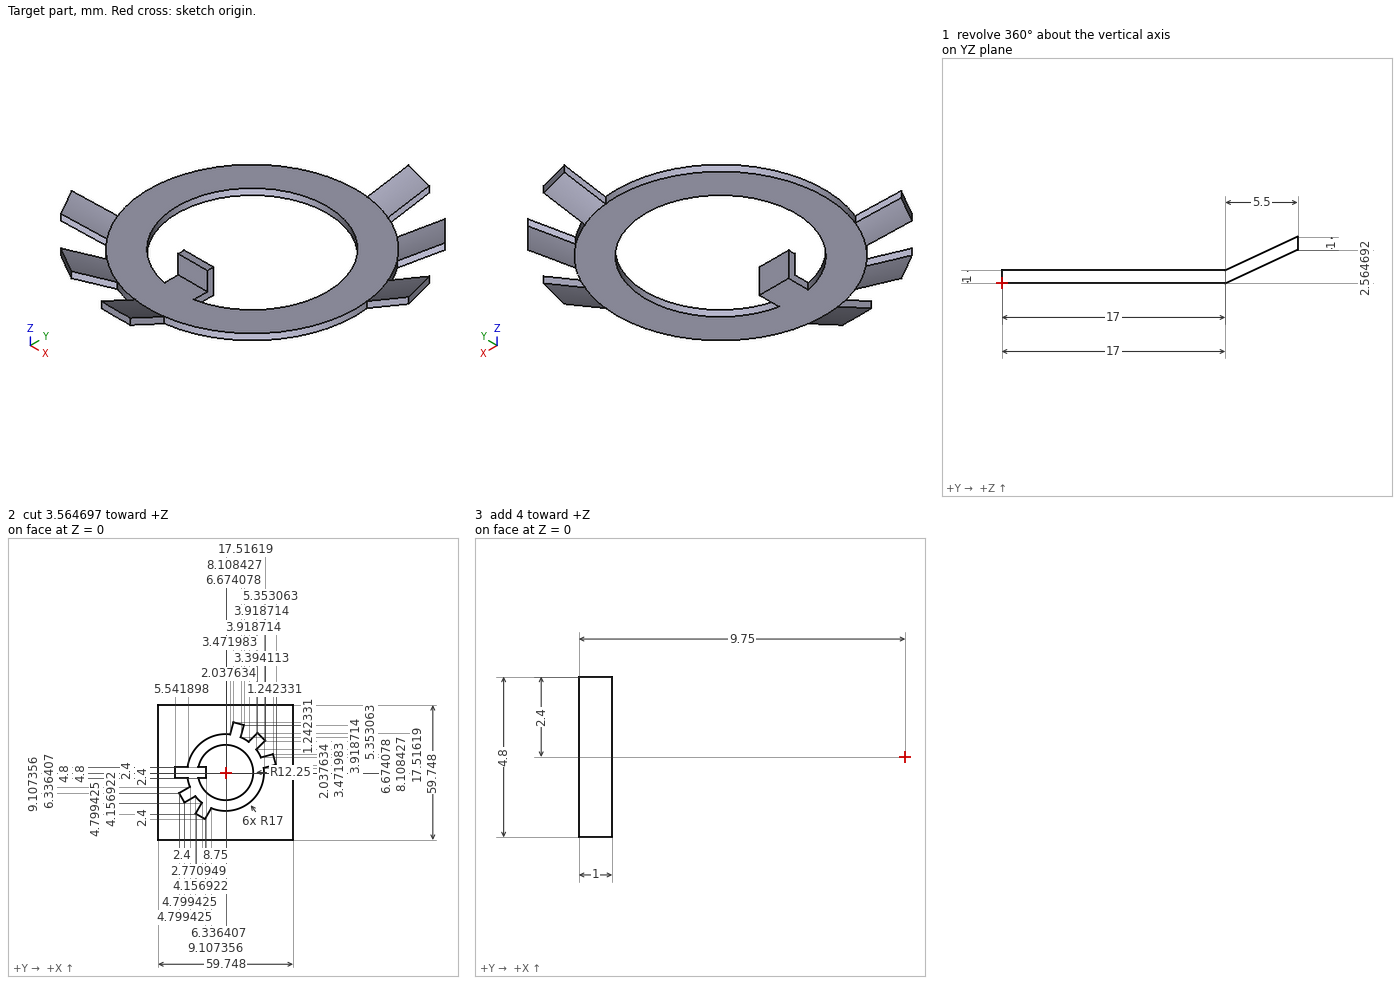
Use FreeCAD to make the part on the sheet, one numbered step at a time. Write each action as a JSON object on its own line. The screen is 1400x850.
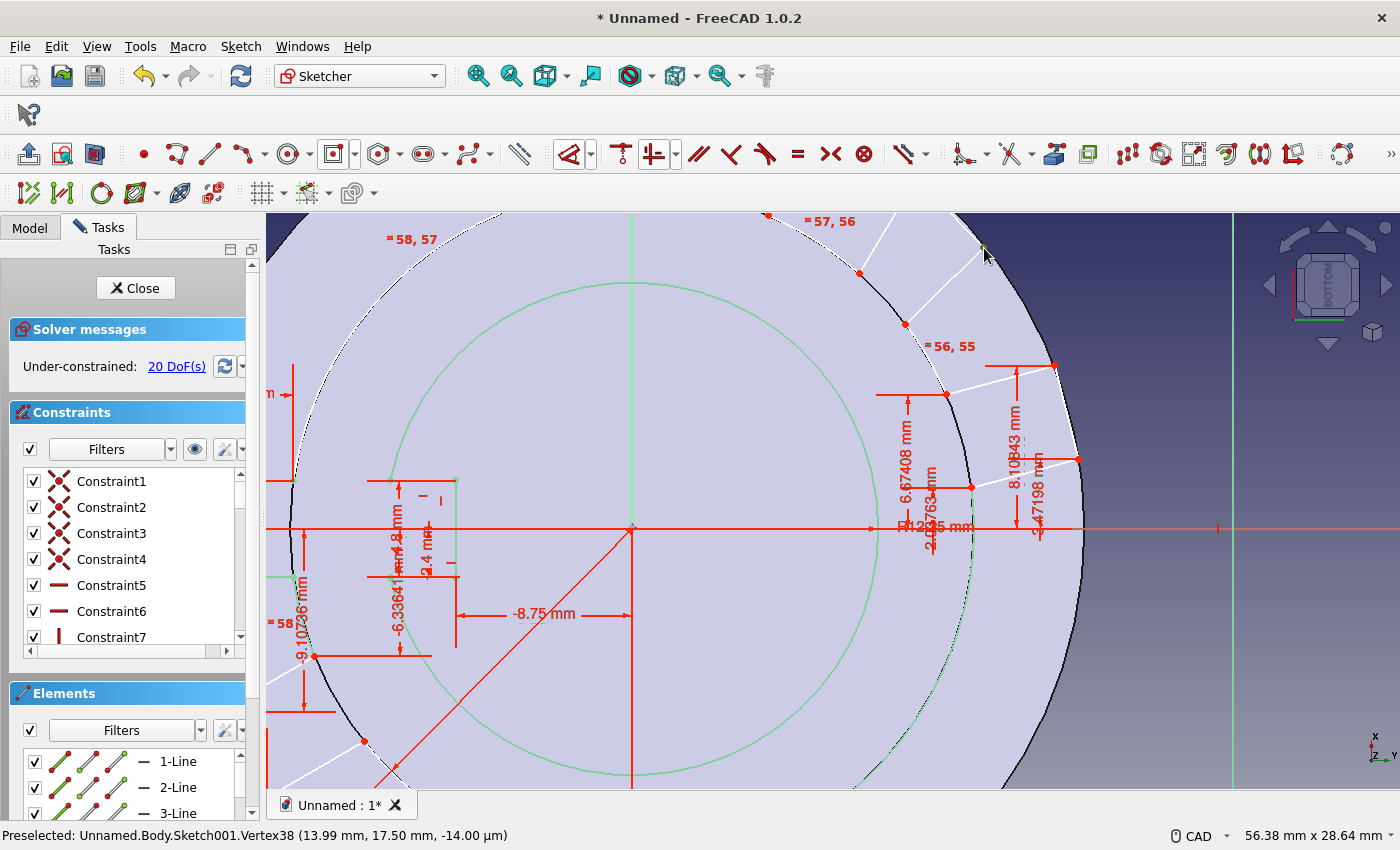
{"action": "left_click", "coordinate": [590, 154]}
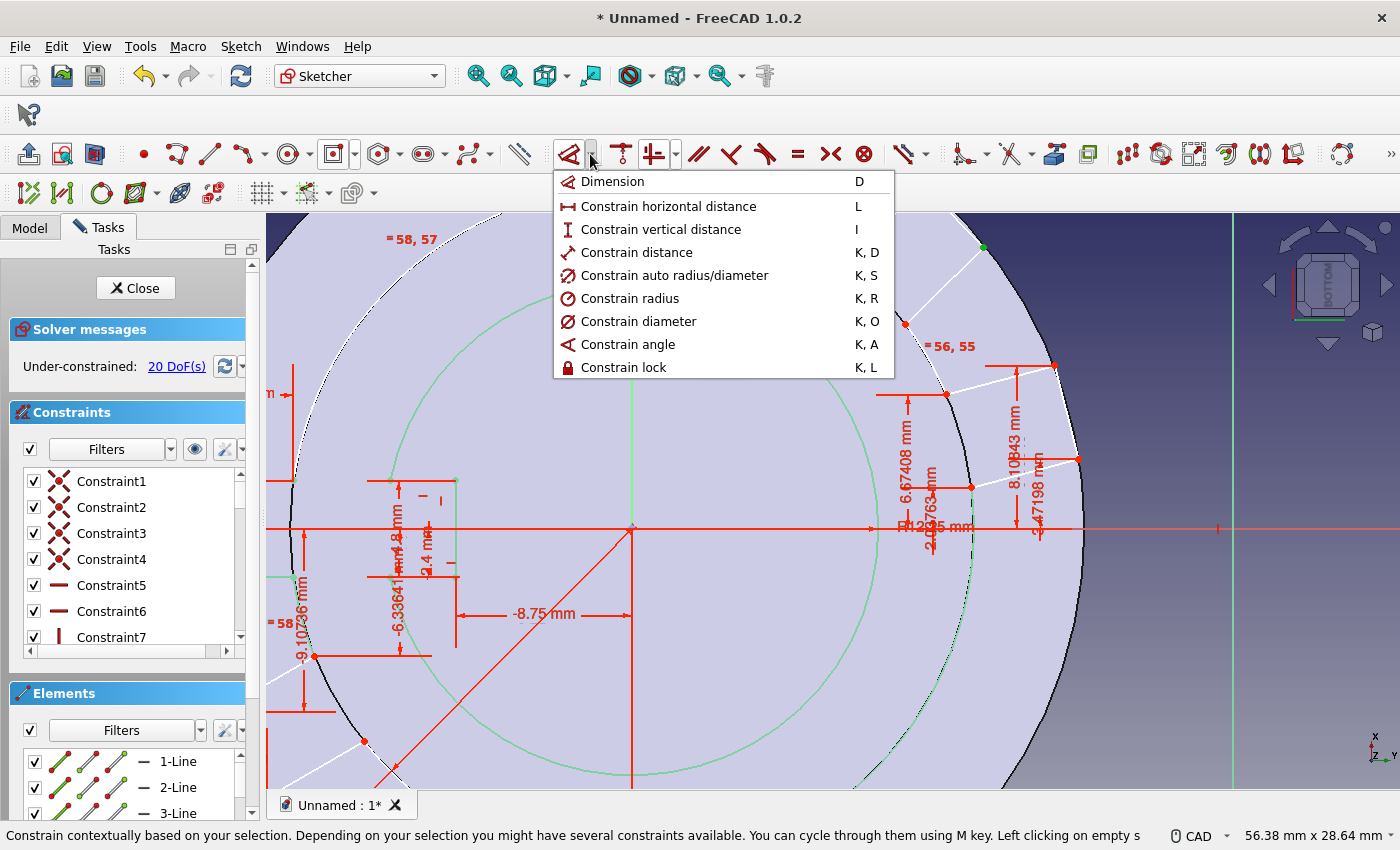
{"action": "left_click", "coordinate": [724, 206]}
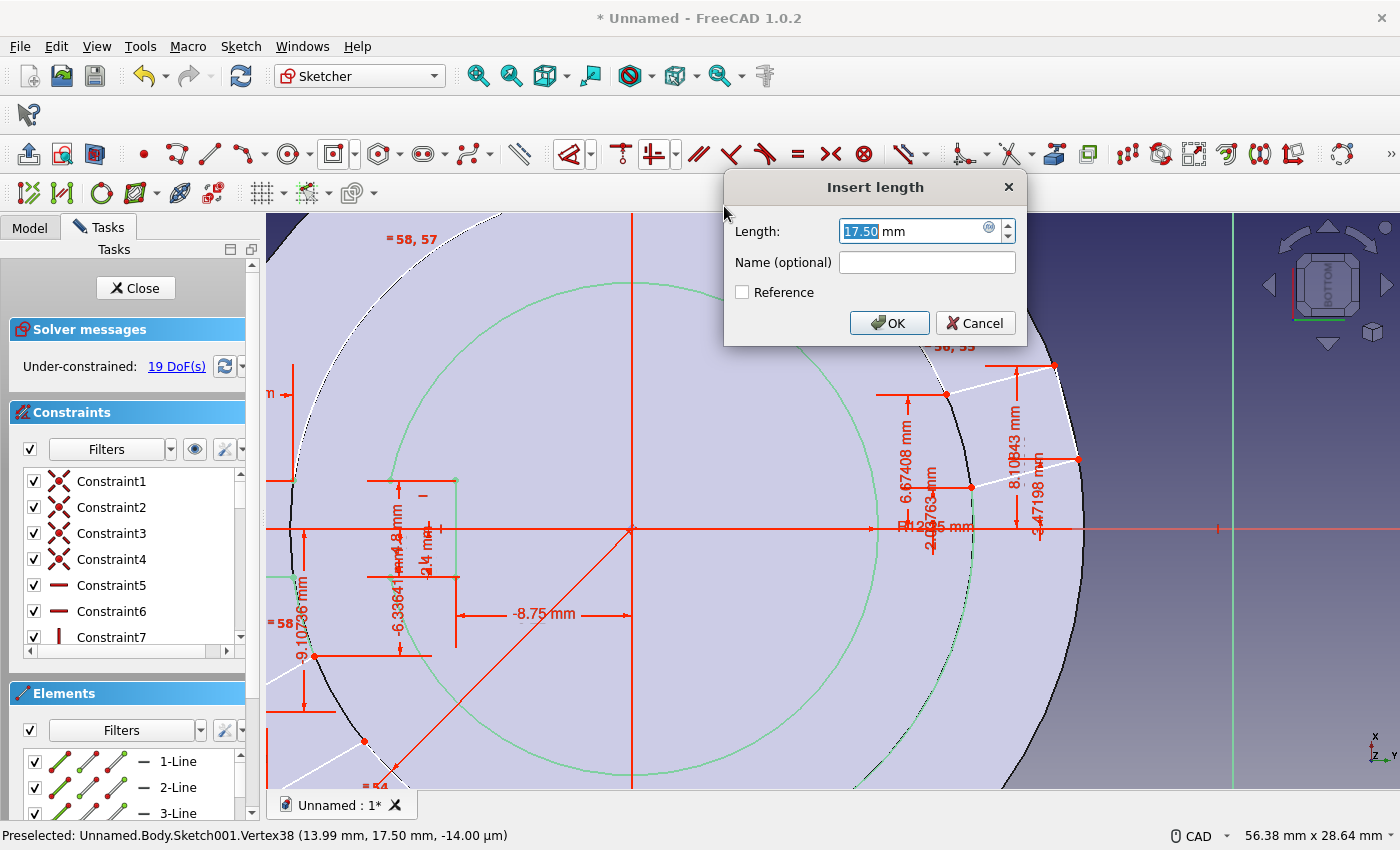
{"action": "type", "text": "17.51619"}
{"action": "key", "text": "Return"}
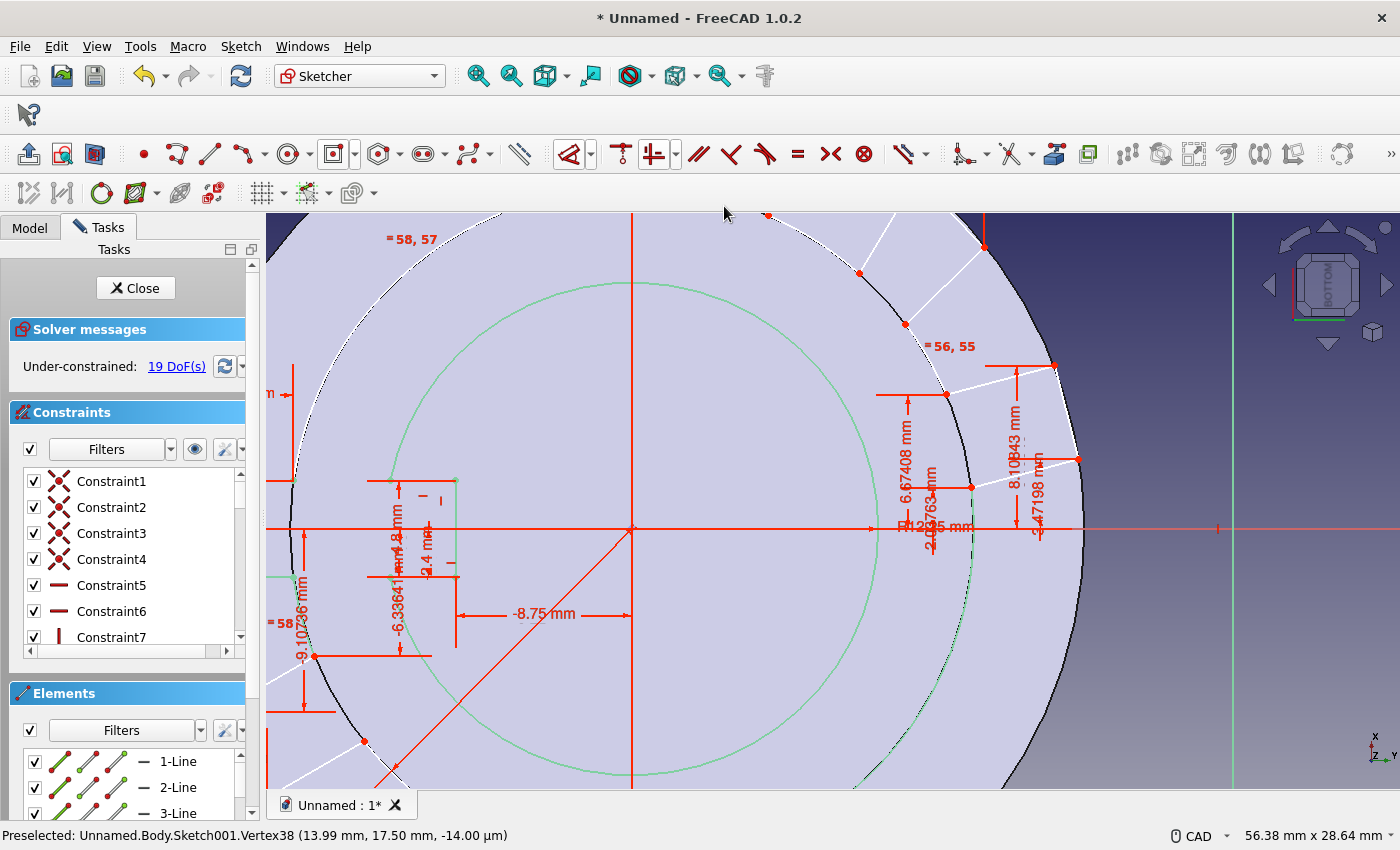
{"action": "scroll", "coordinate": [822, 489], "scroll_direction": "down", "scroll_amount": 6}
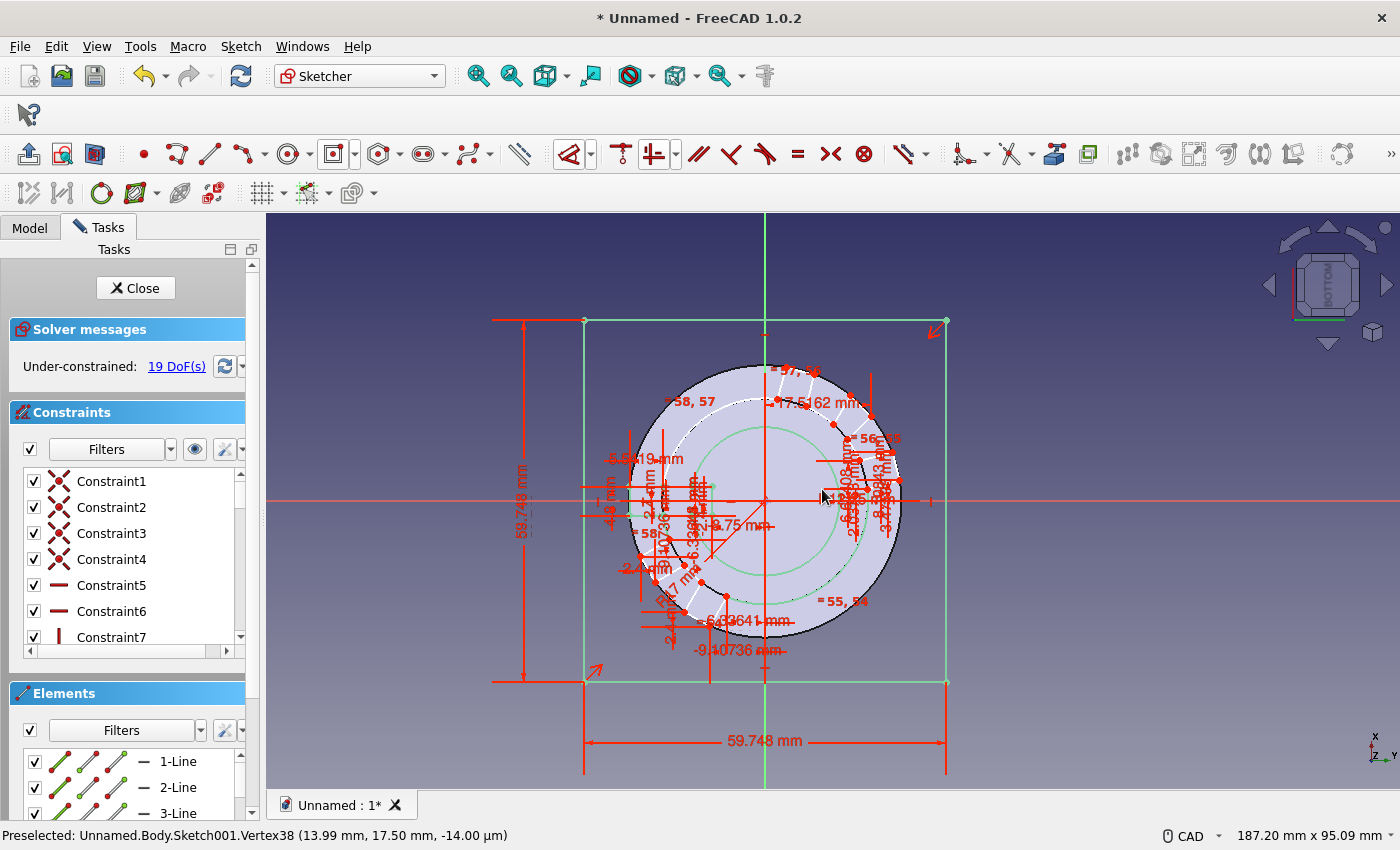
{"action": "left_click", "coordinate": [851, 396]}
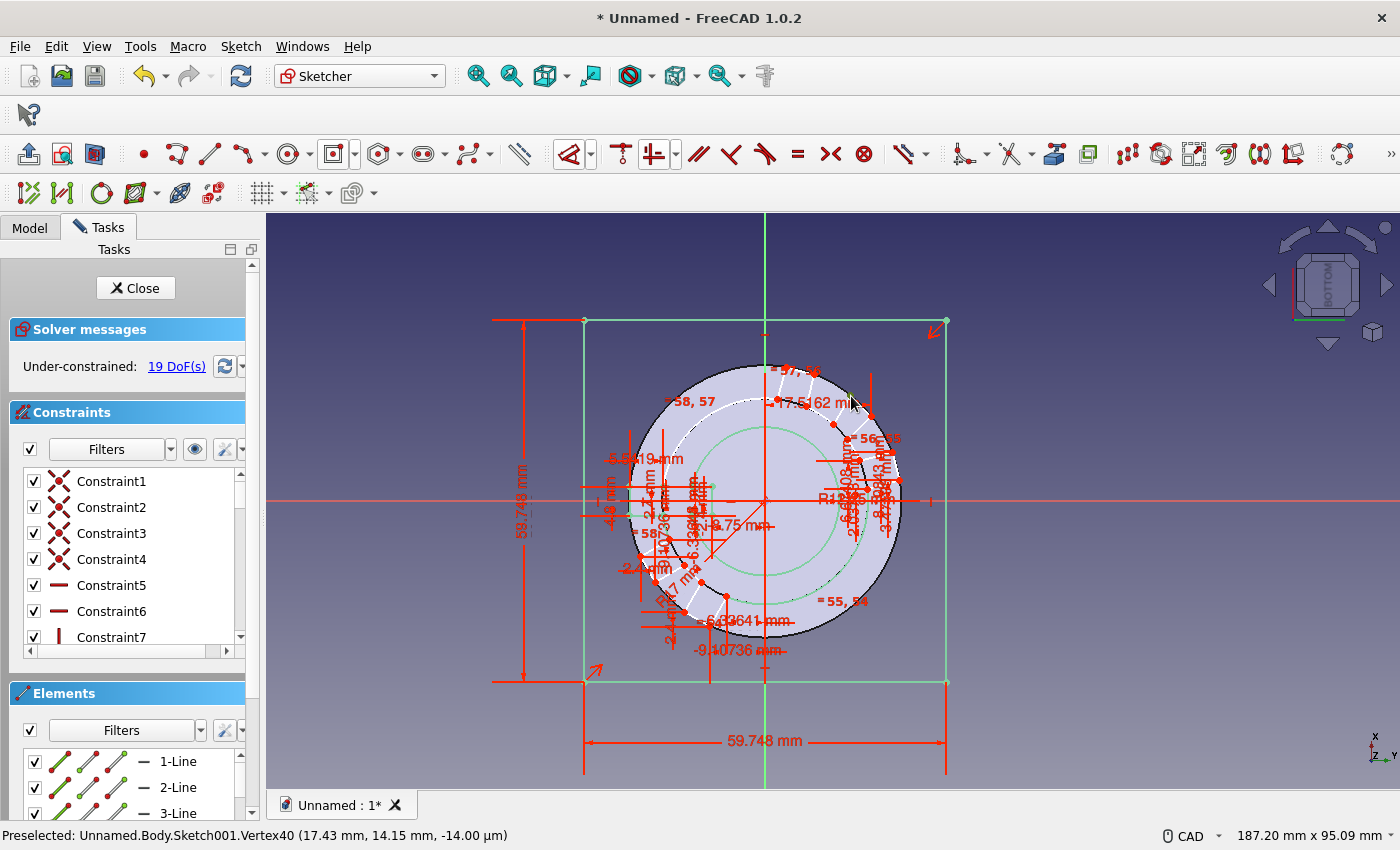
{"action": "left_click", "coordinate": [590, 154]}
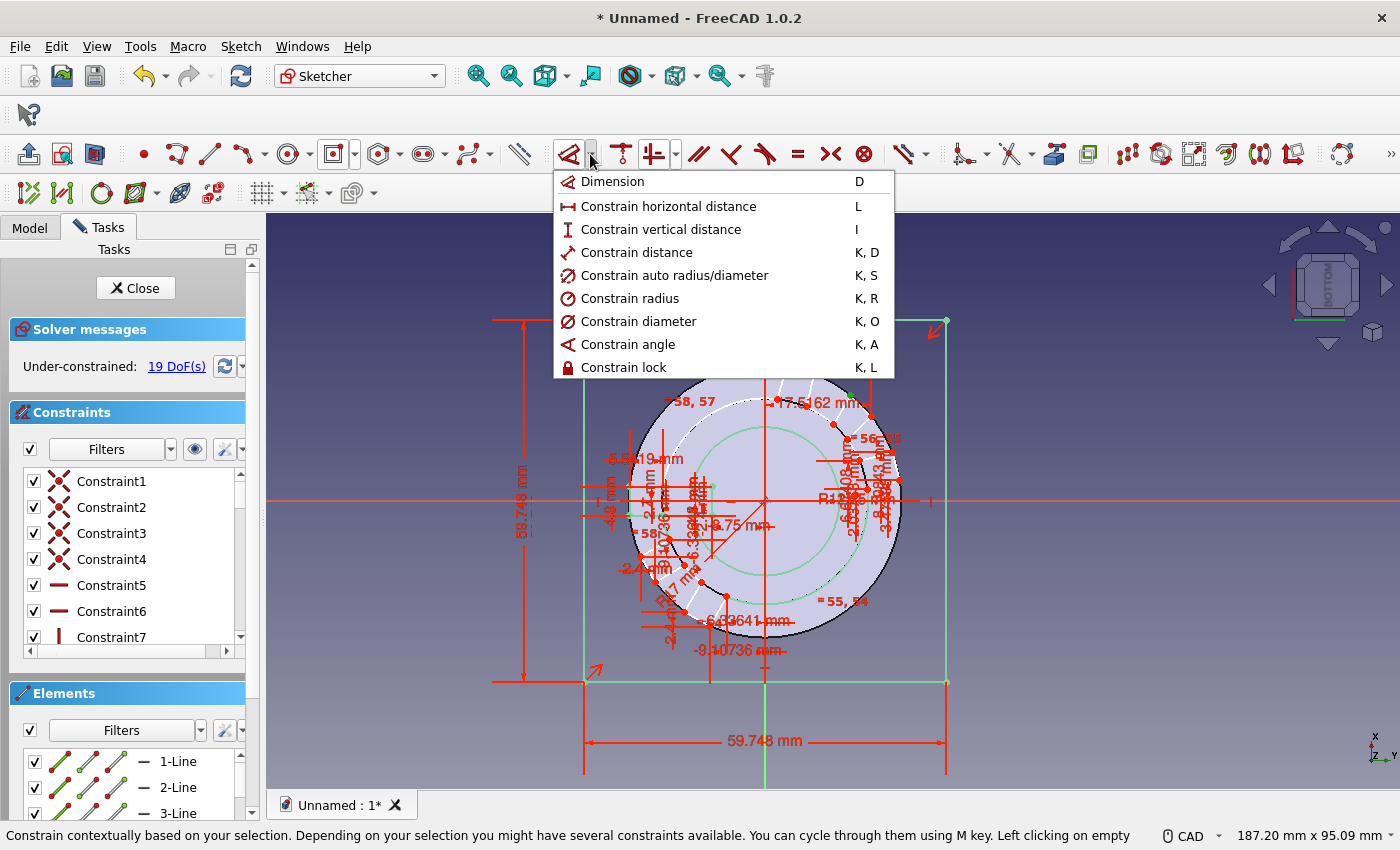
{"action": "left_click", "coordinate": [724, 230]}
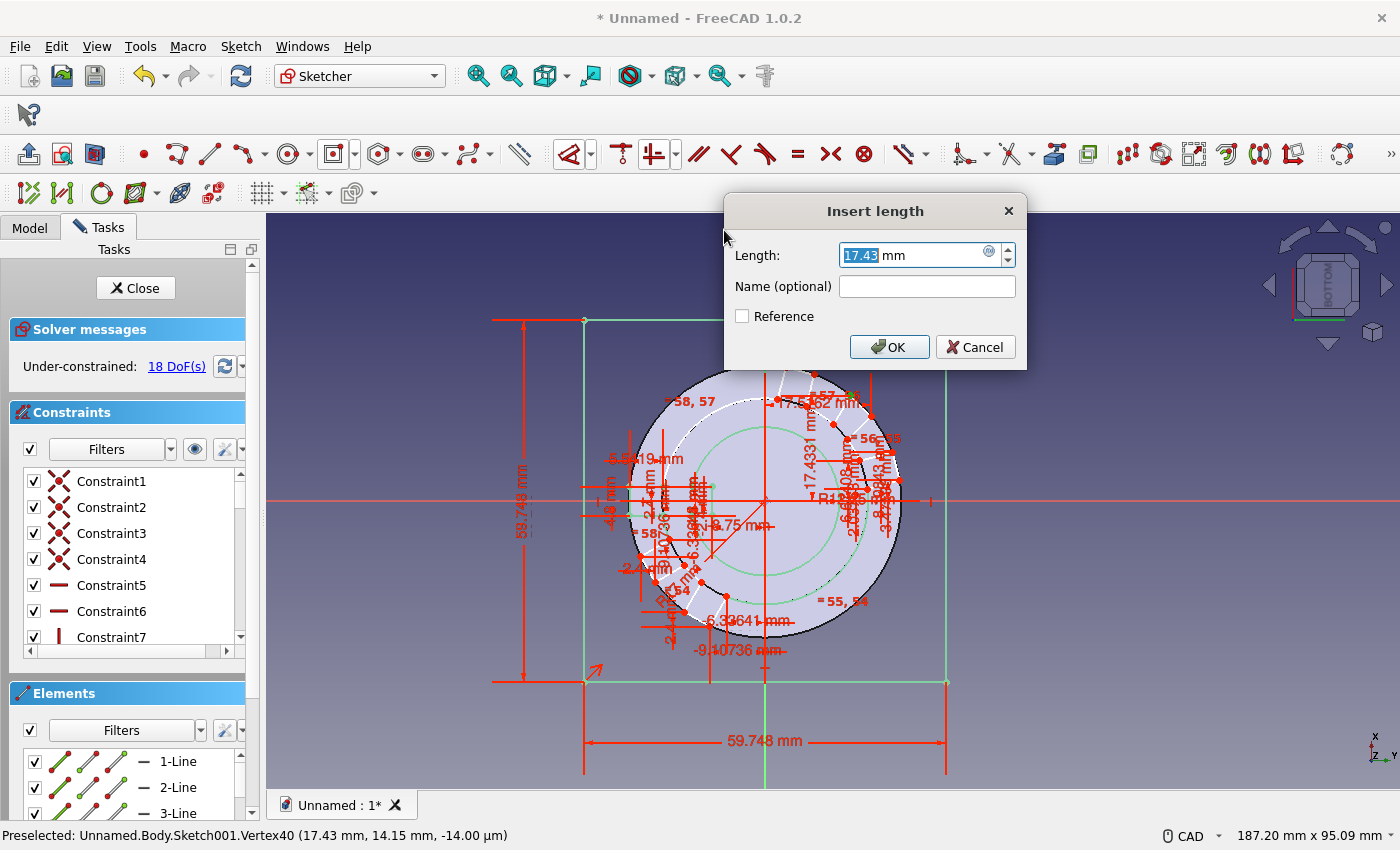
{"action": "type", "text": "17.51619"}
{"action": "key", "text": "Return"}